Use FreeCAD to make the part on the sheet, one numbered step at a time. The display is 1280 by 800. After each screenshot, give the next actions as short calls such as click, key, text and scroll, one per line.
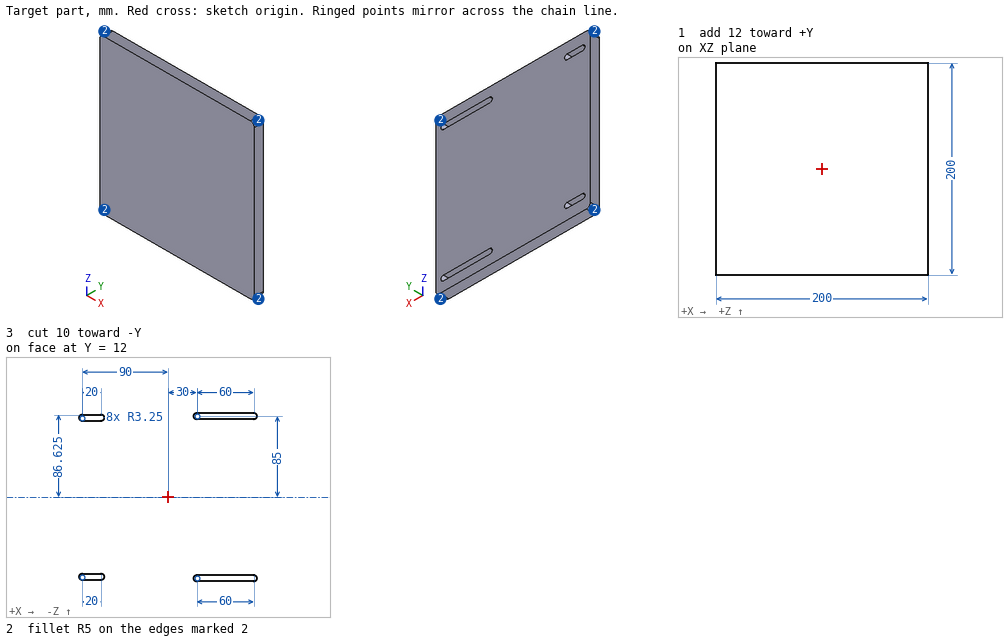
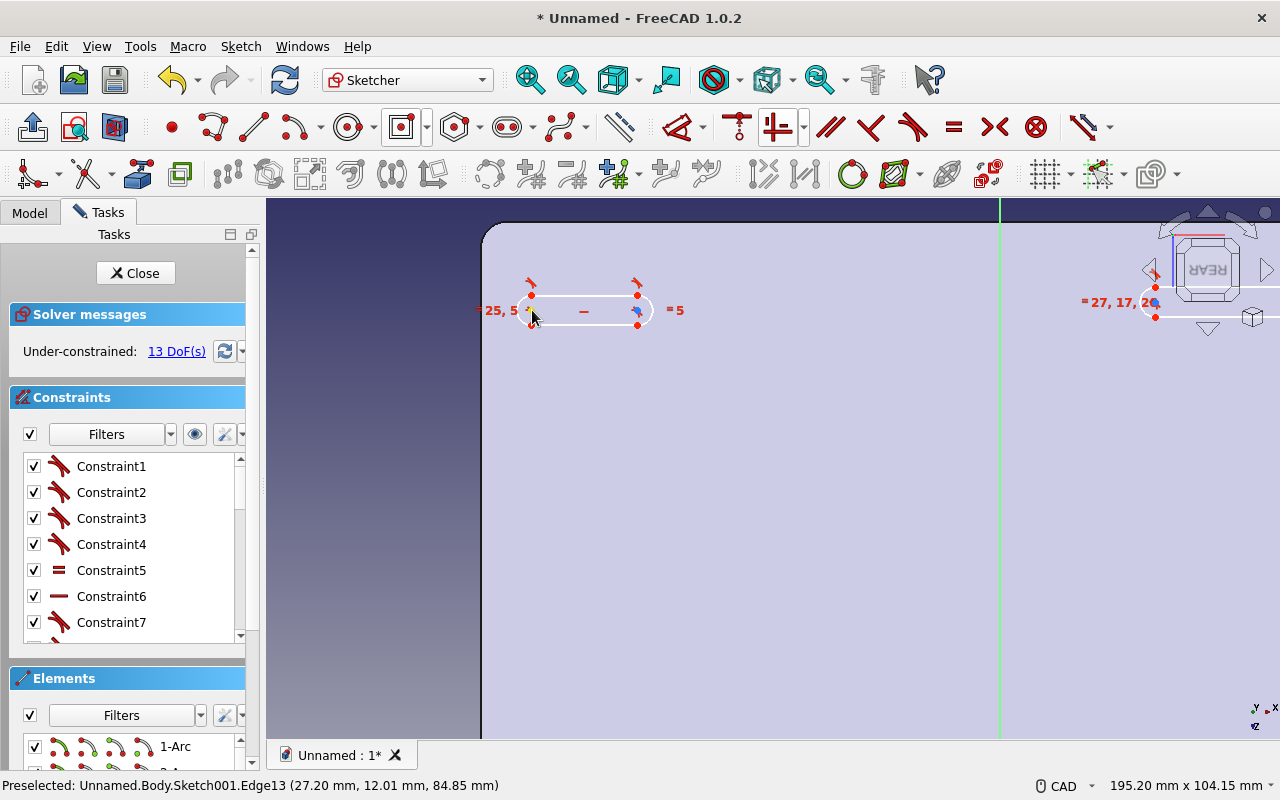
click(532, 310)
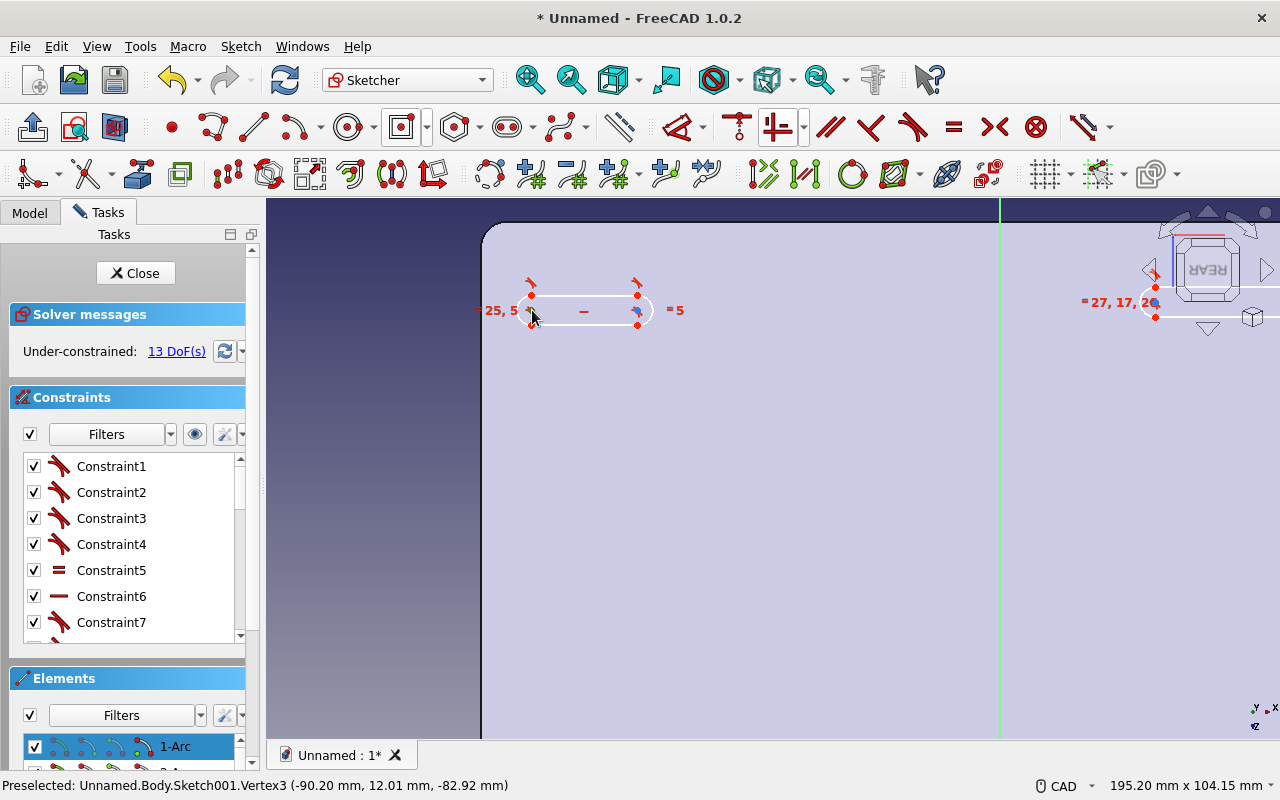
scroll(532, 310, down, 5)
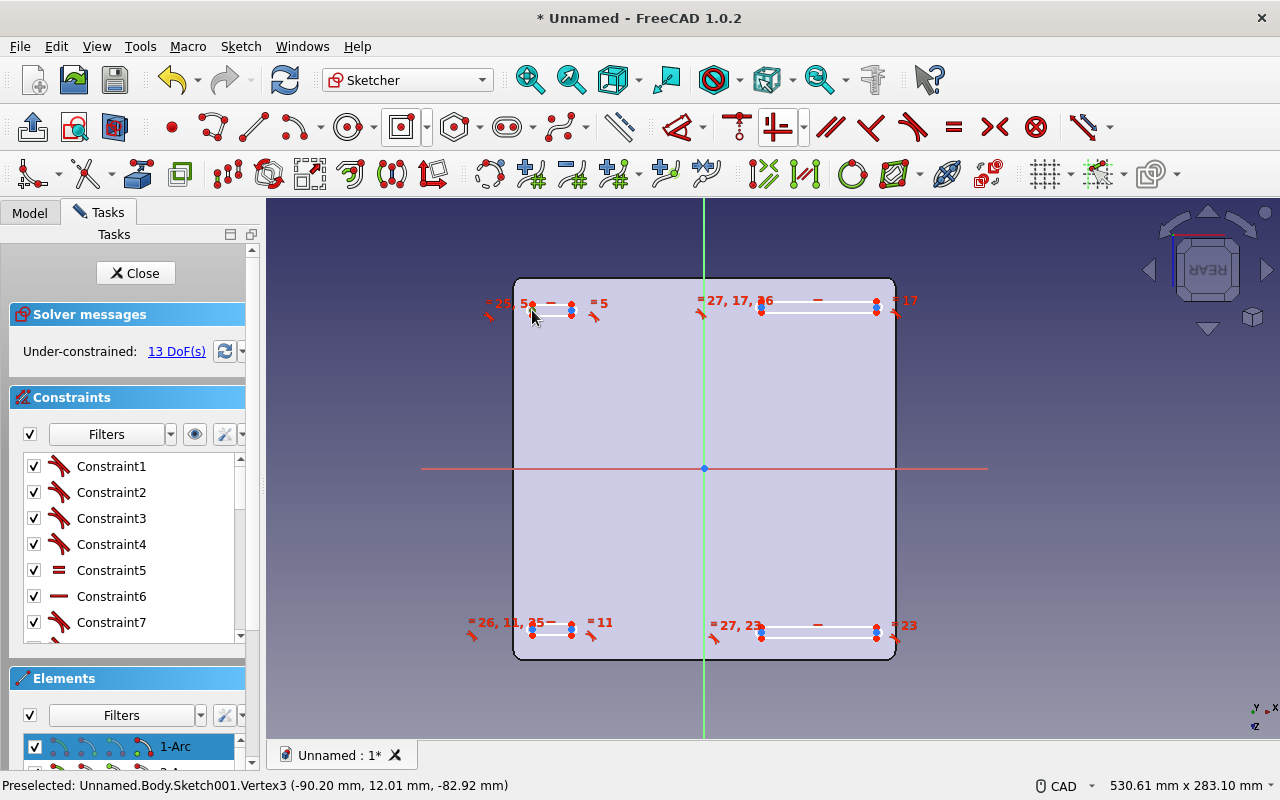
scroll(532, 630, up, 5)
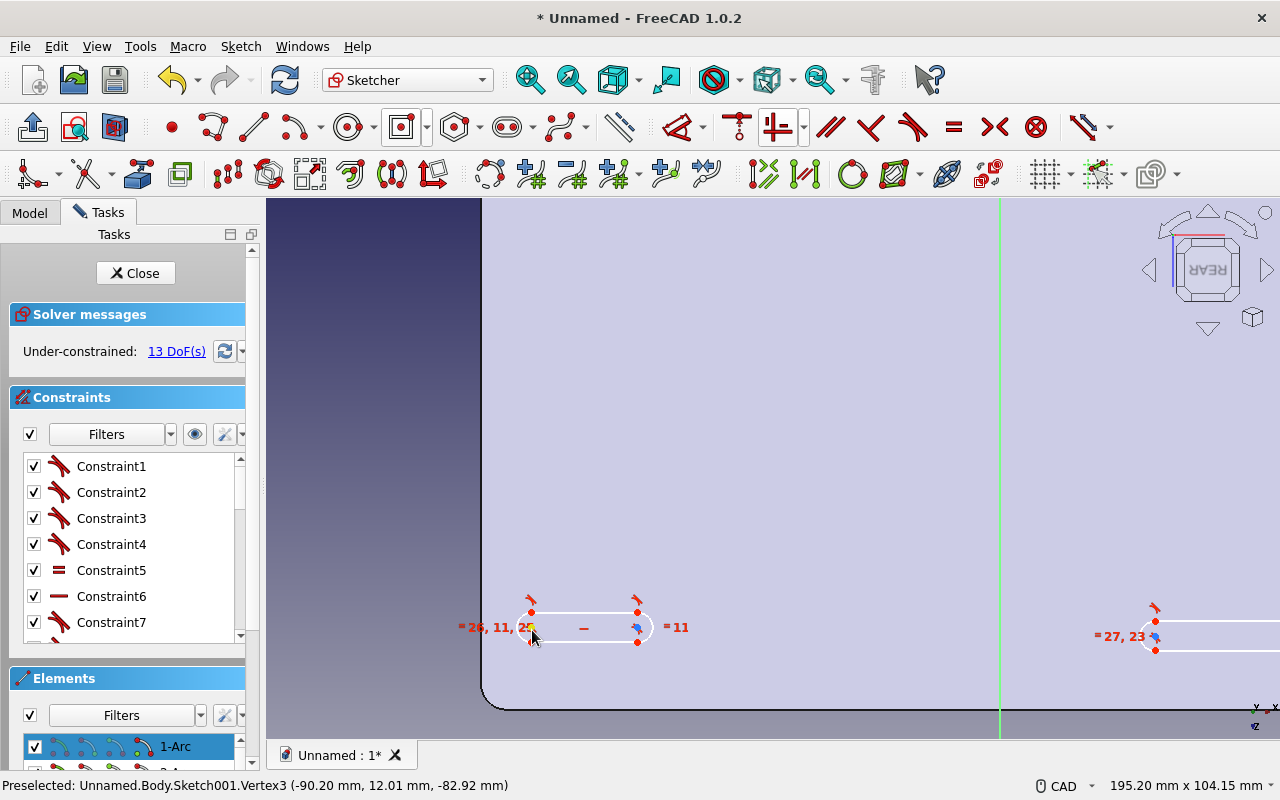
click(532, 628)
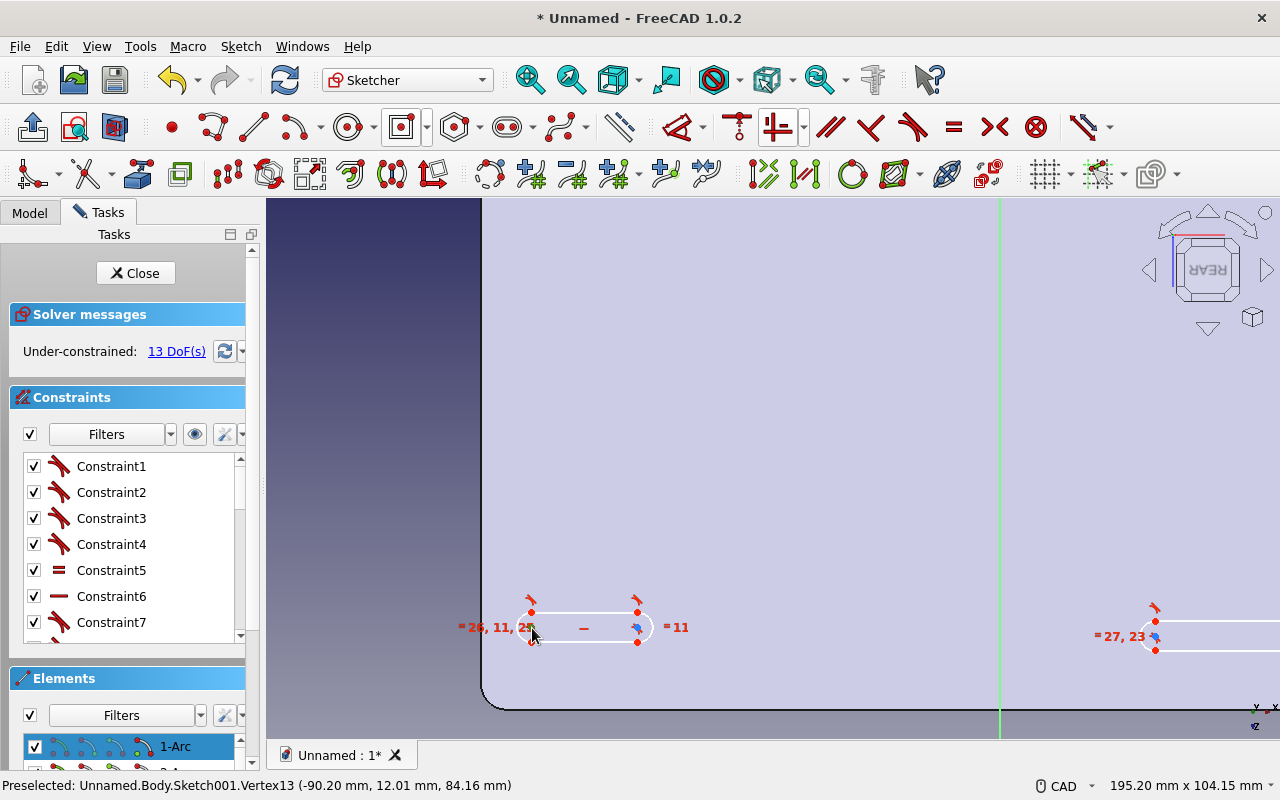
scroll(532, 630, down, 5)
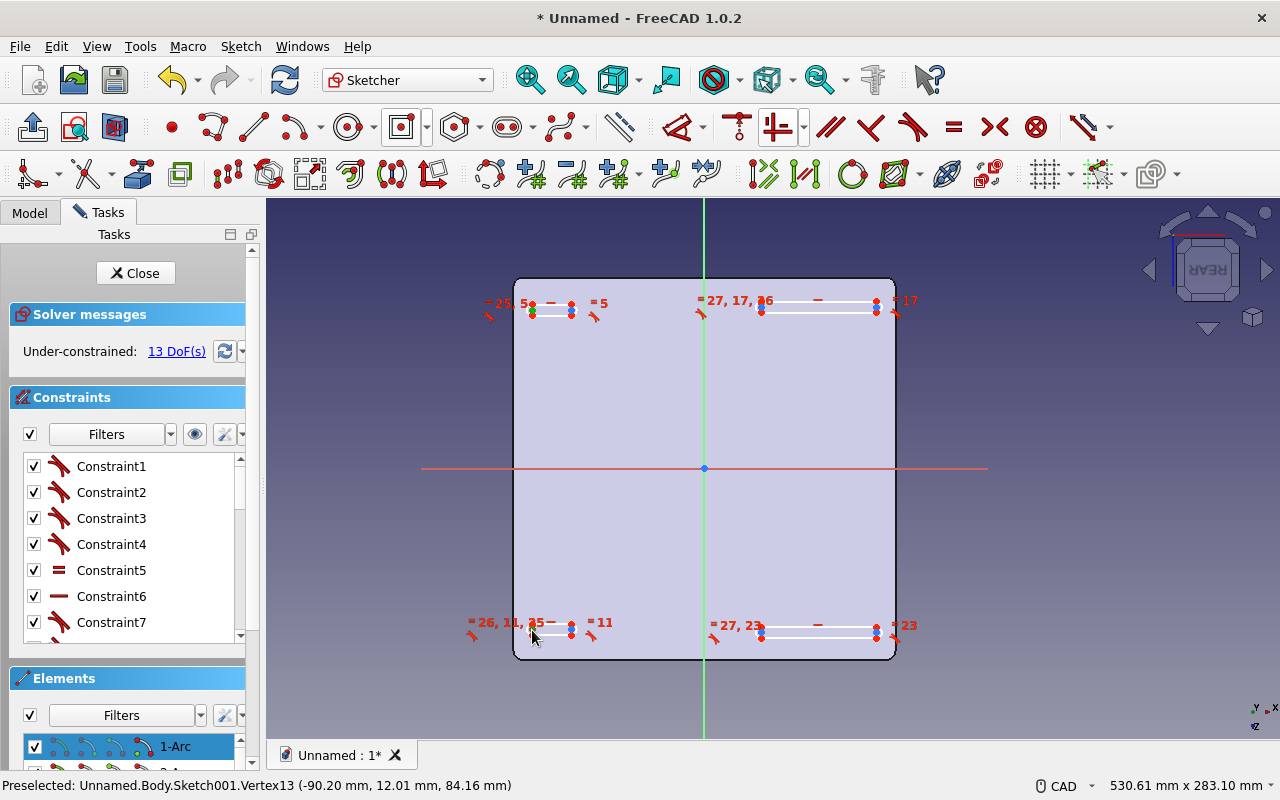
click(470, 469)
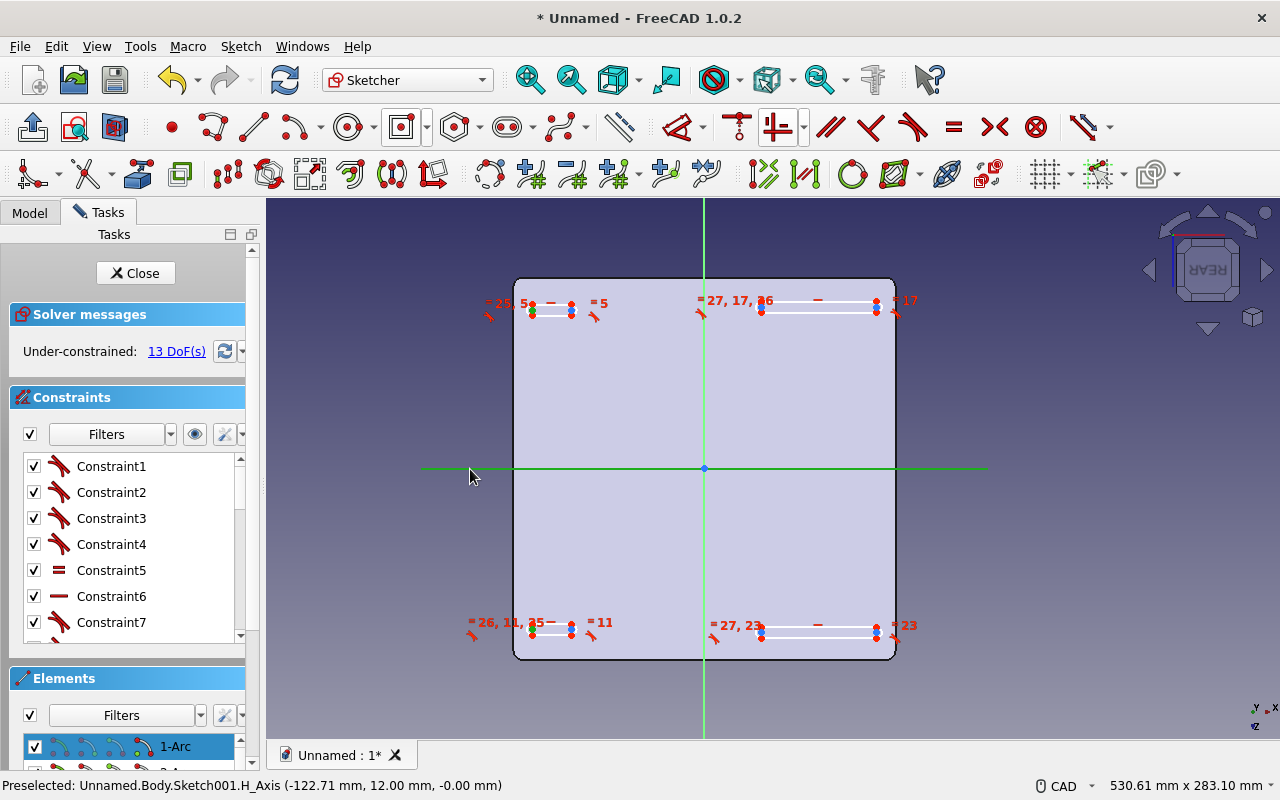
click(995, 128)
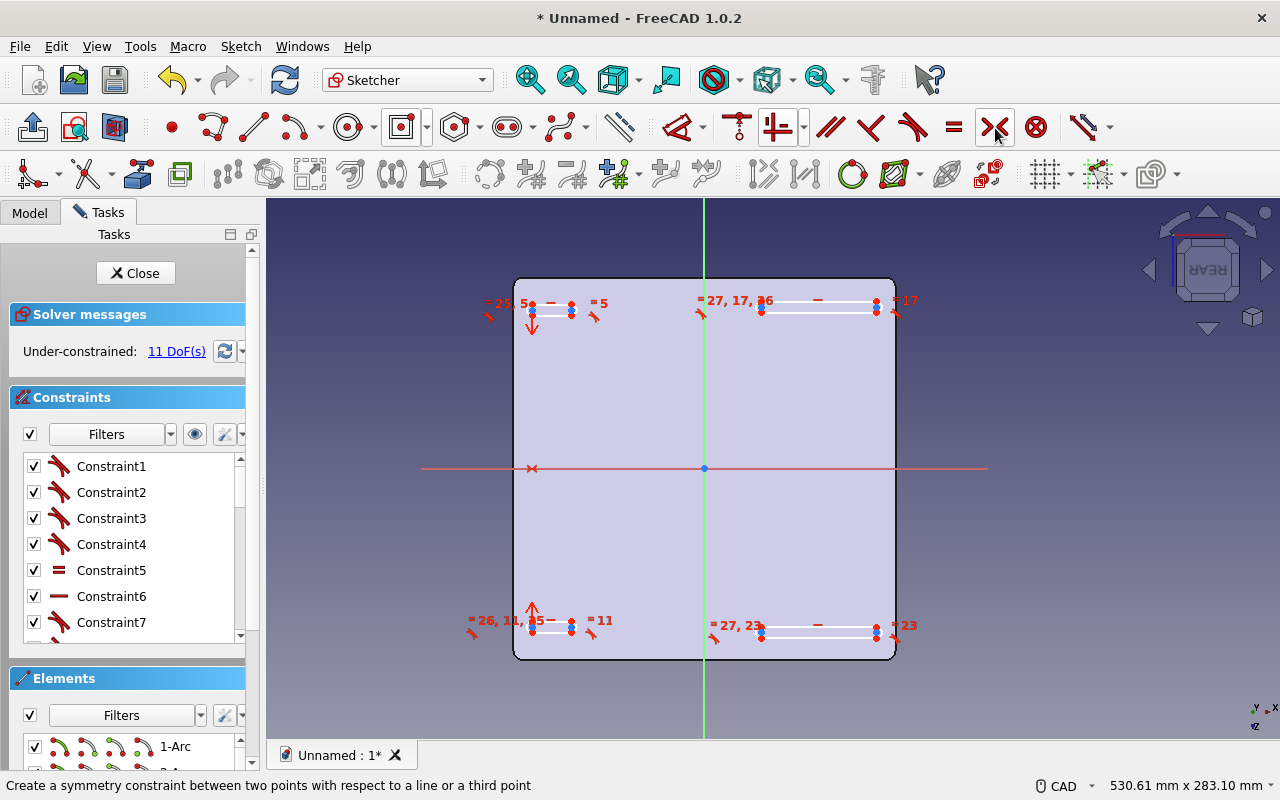
scroll(761, 307, up, 5)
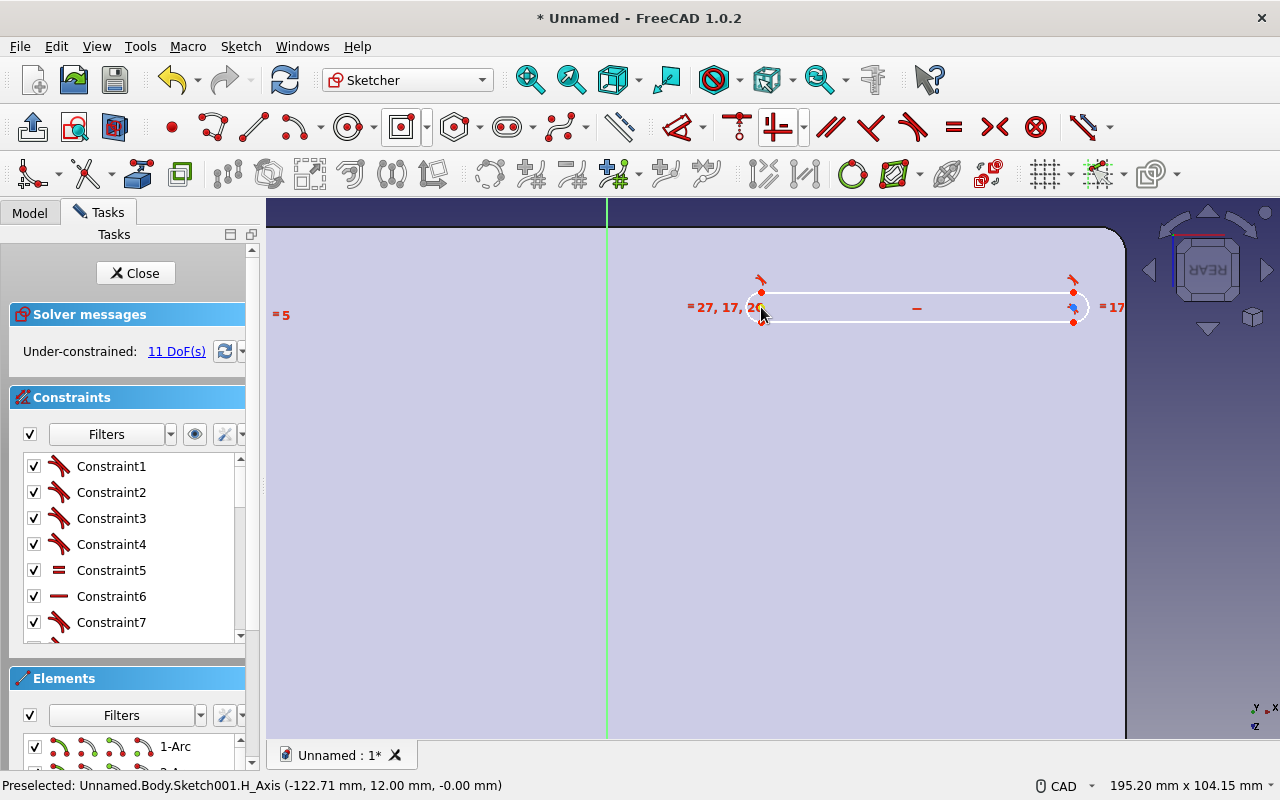
click(761, 307)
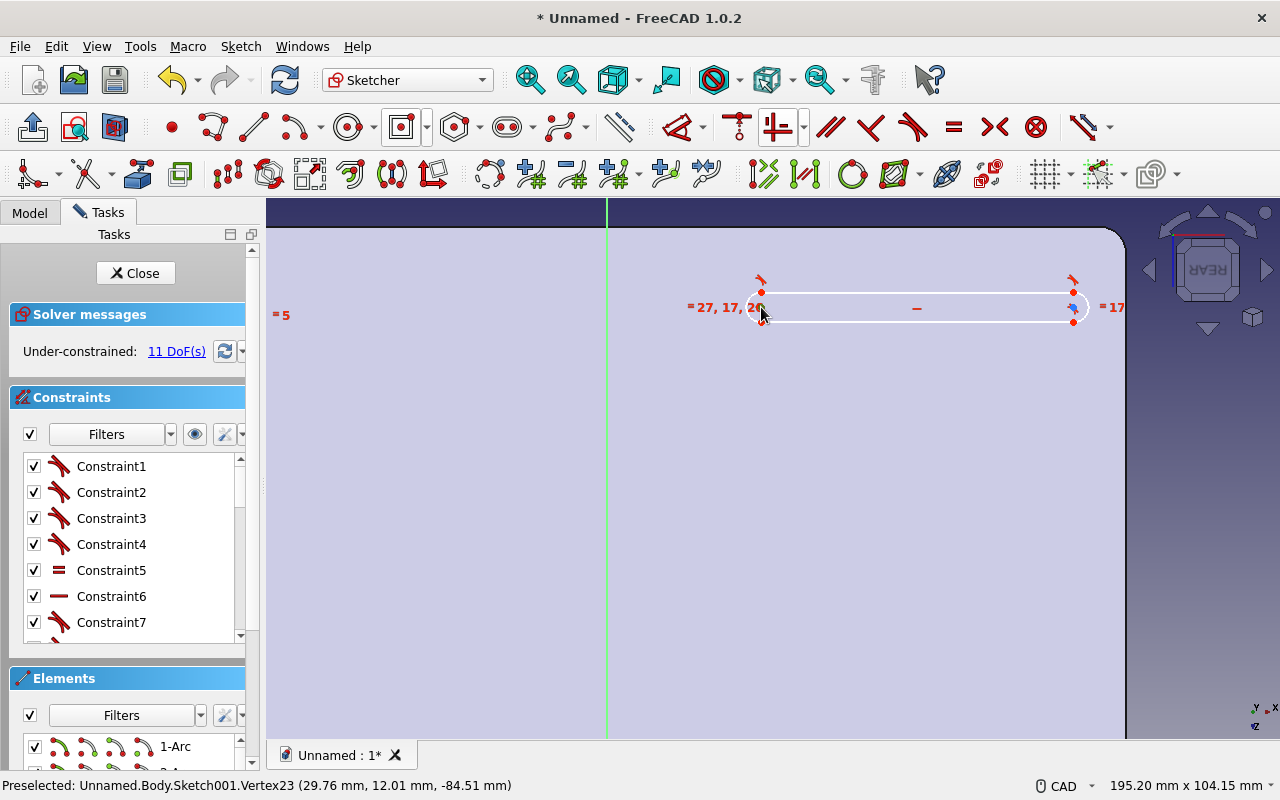
scroll(761, 307, down, 5)